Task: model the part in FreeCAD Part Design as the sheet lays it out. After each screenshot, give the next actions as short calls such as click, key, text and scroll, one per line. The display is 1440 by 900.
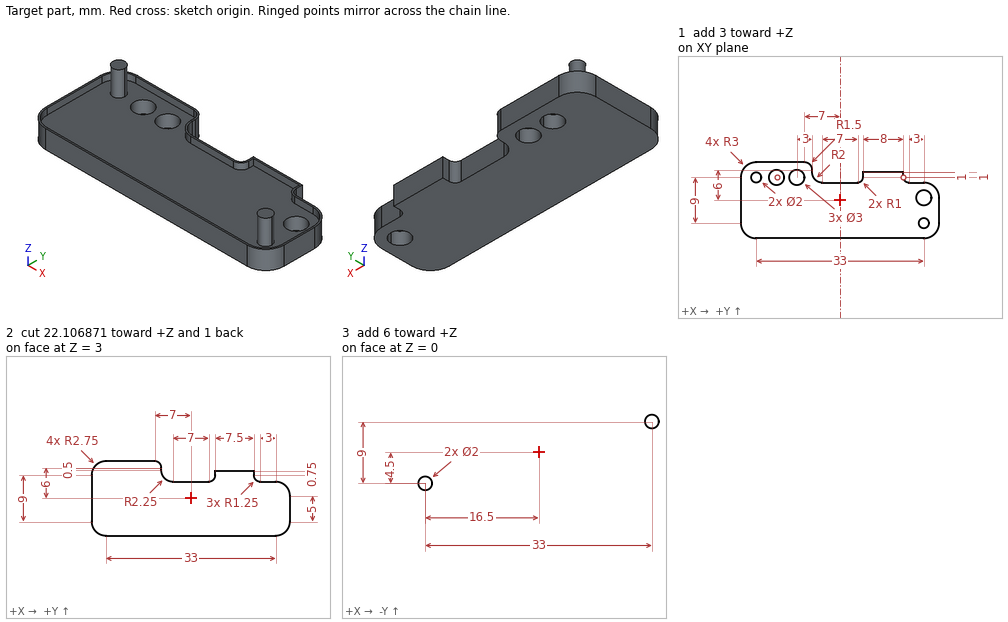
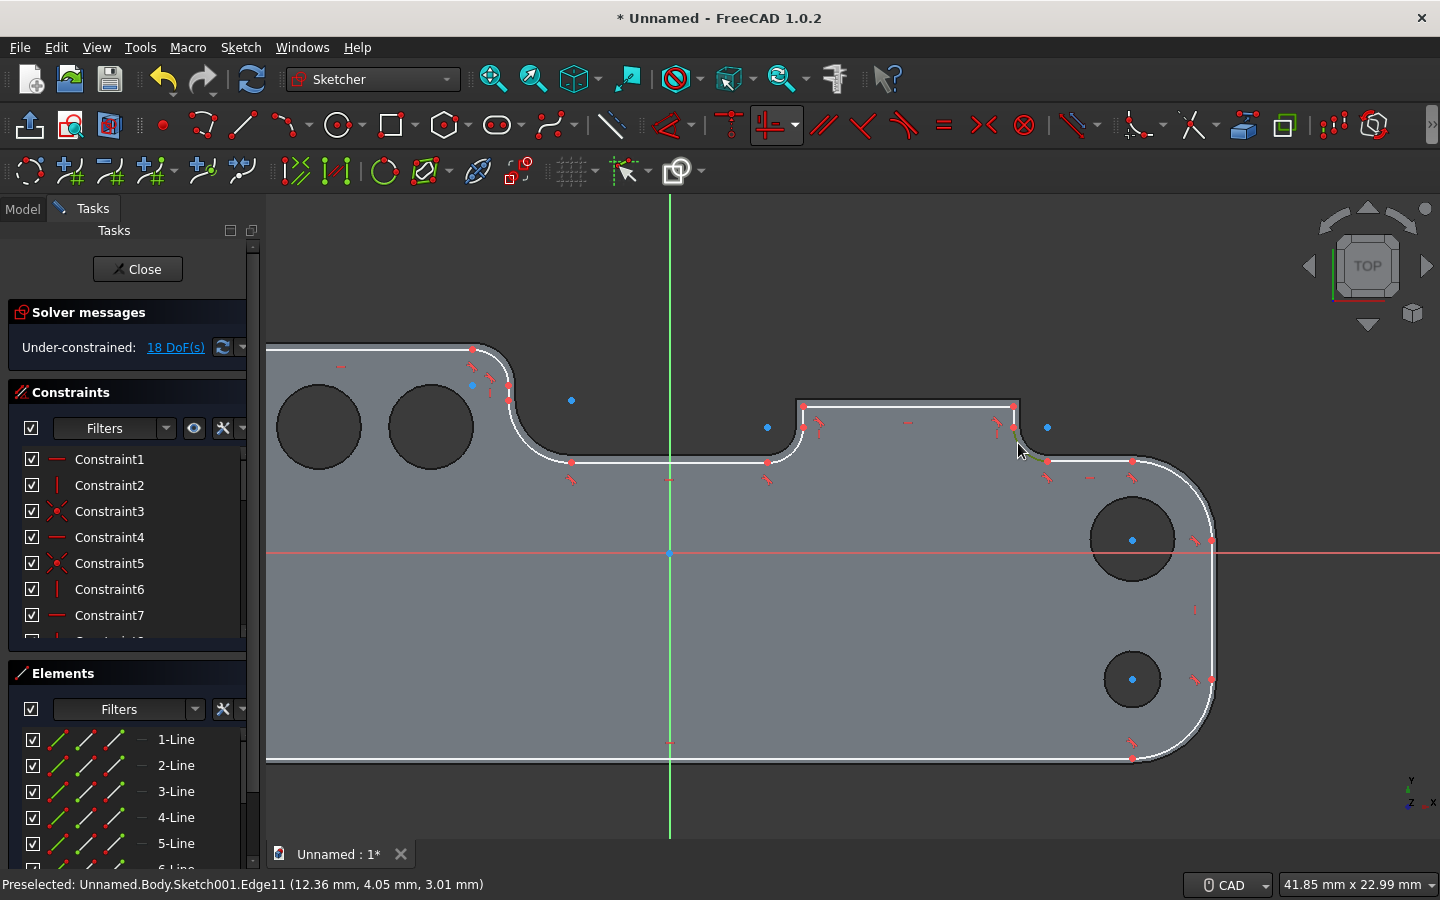
click(784, 459)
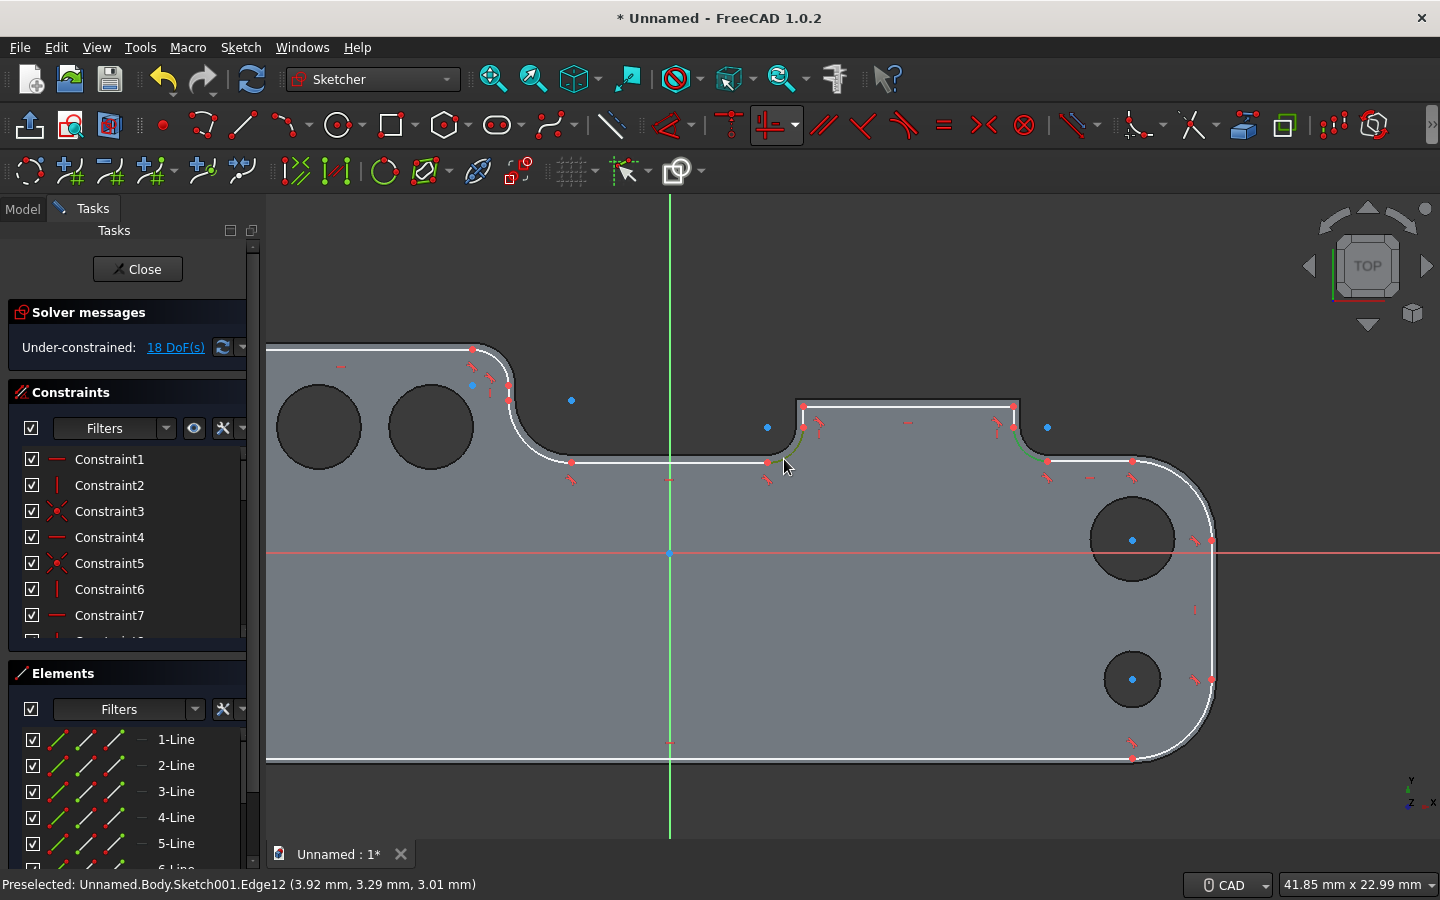
click(505, 370)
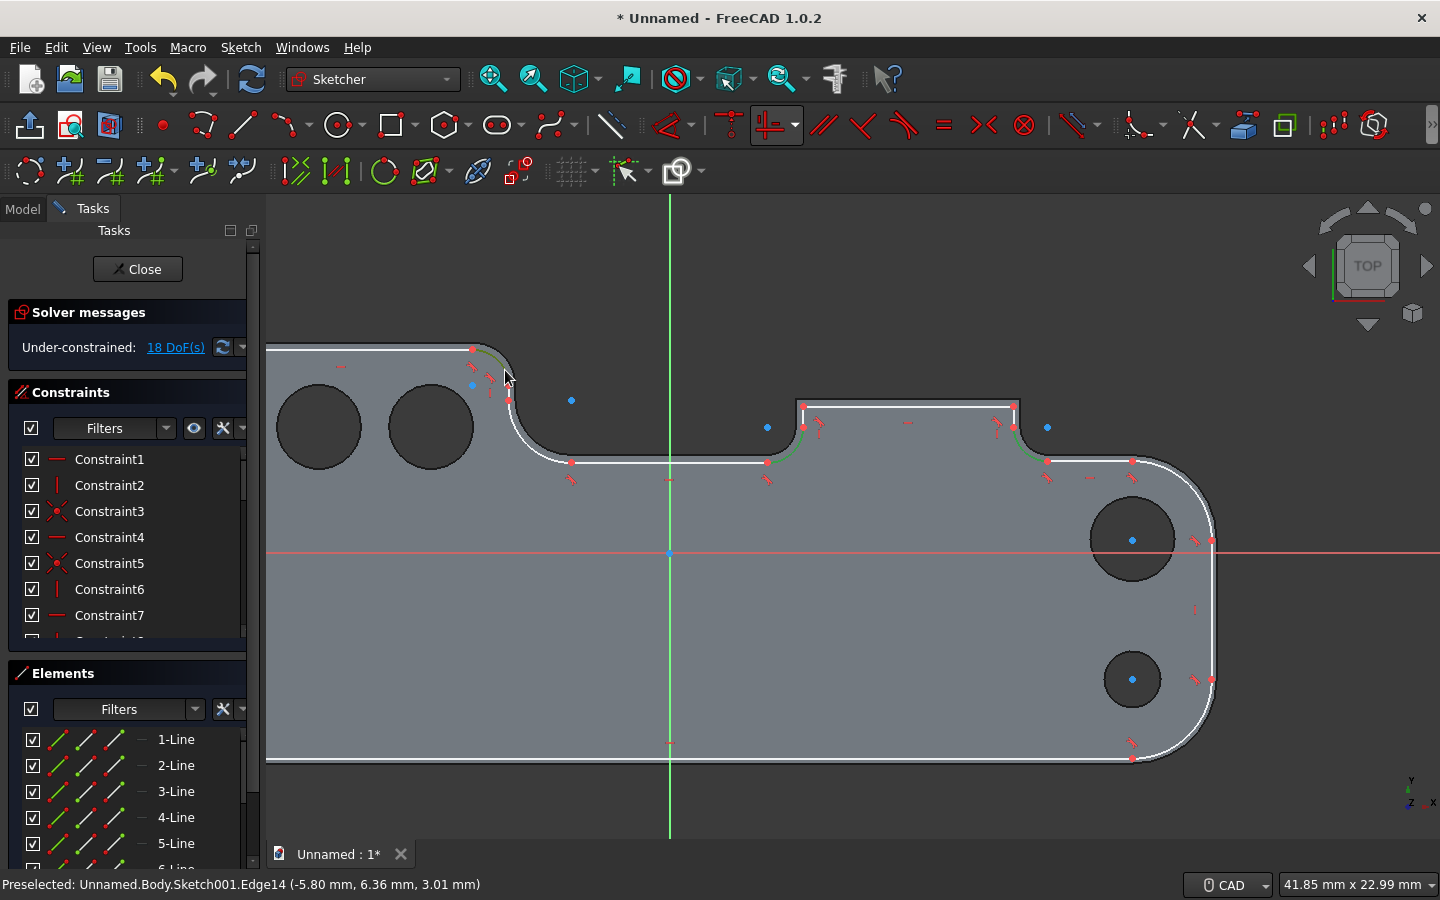
key(e)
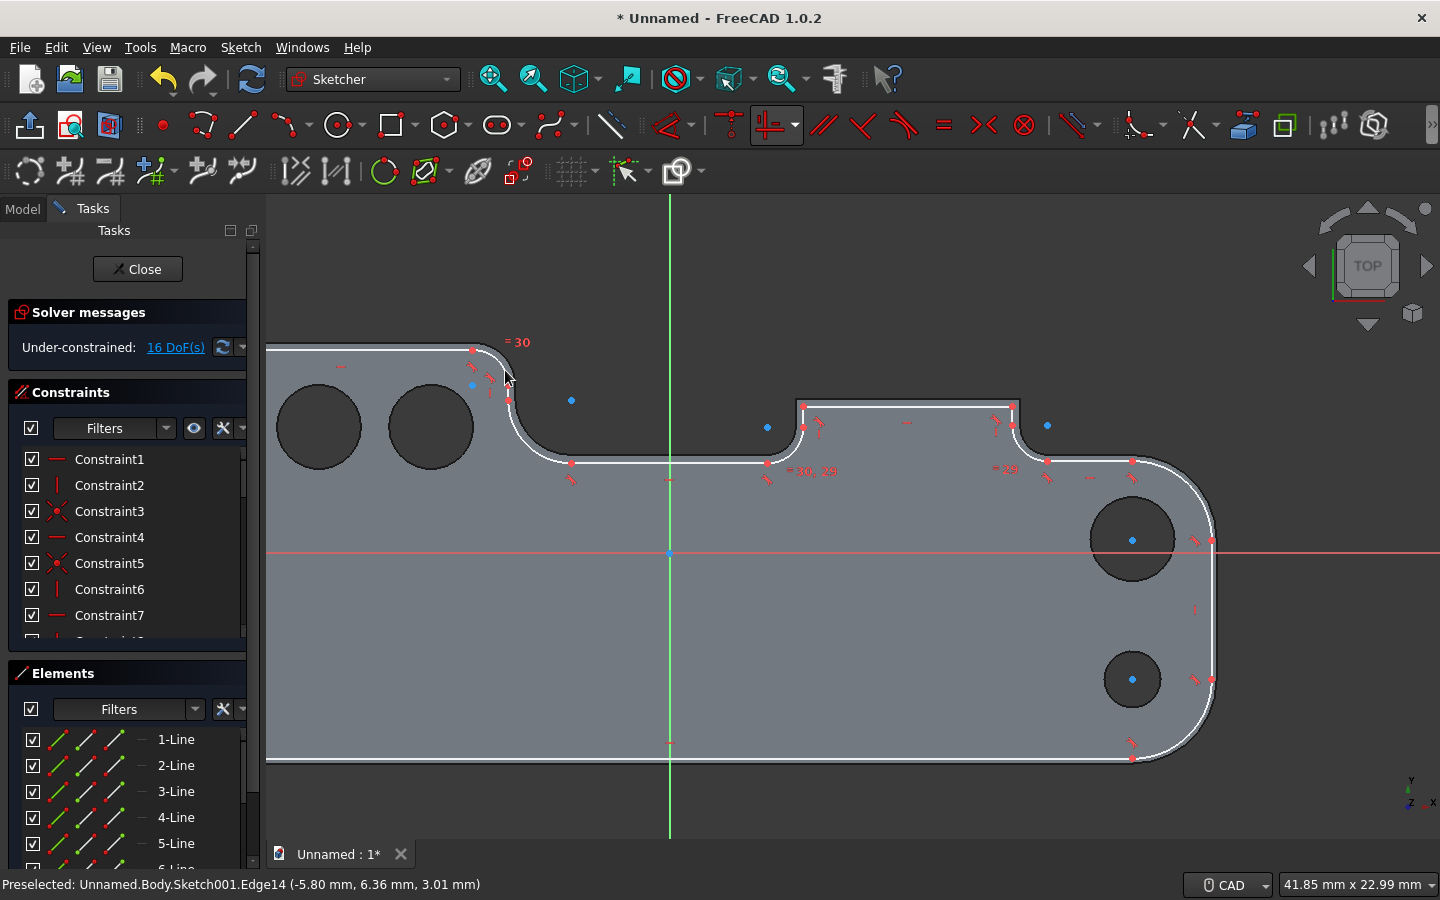
scroll(1018, 442, down, 2)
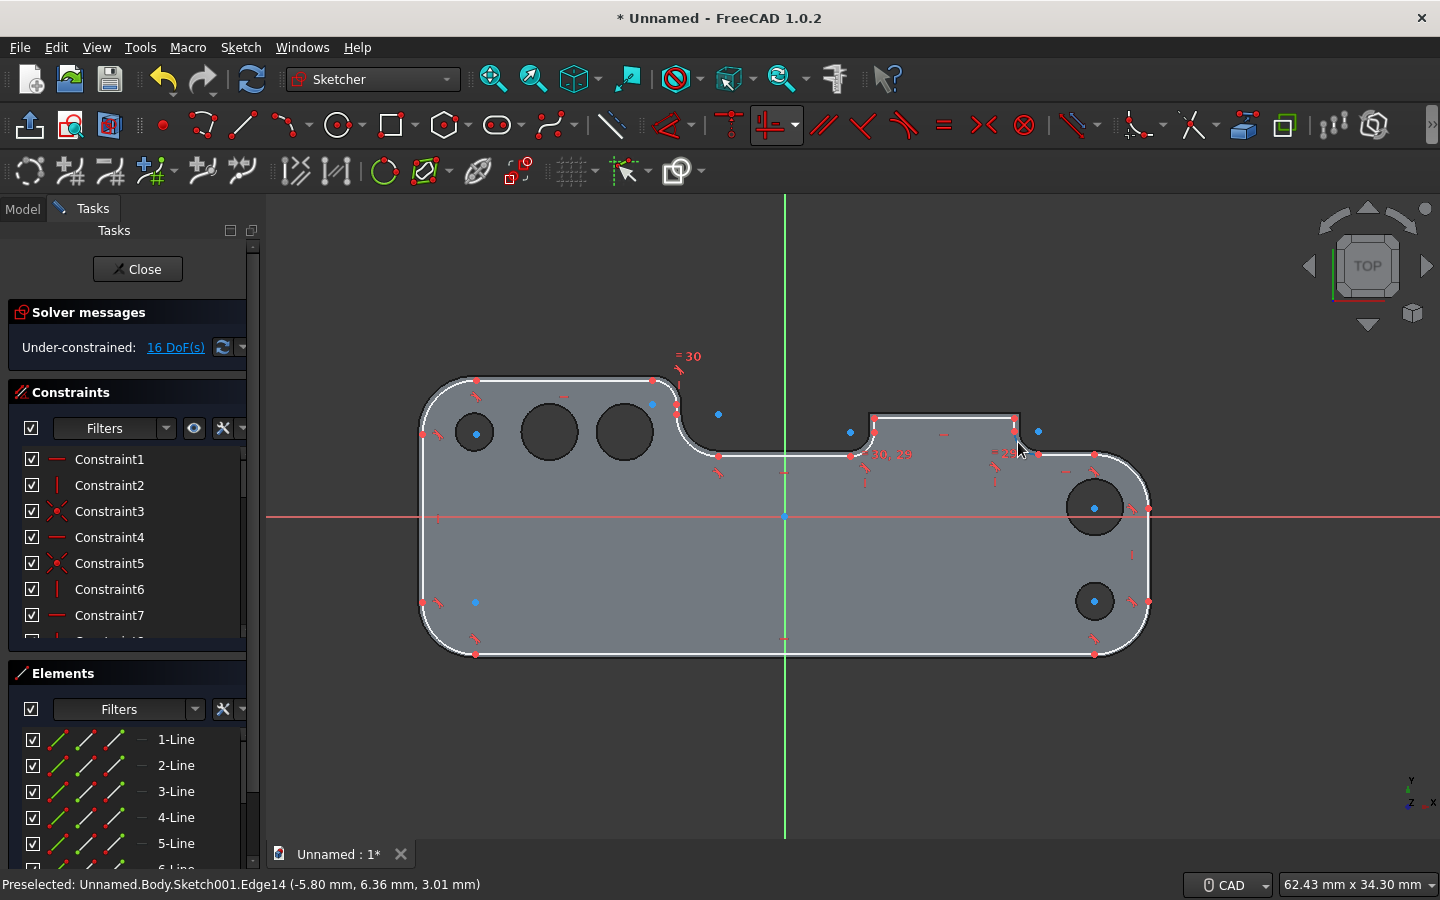
click(452, 386)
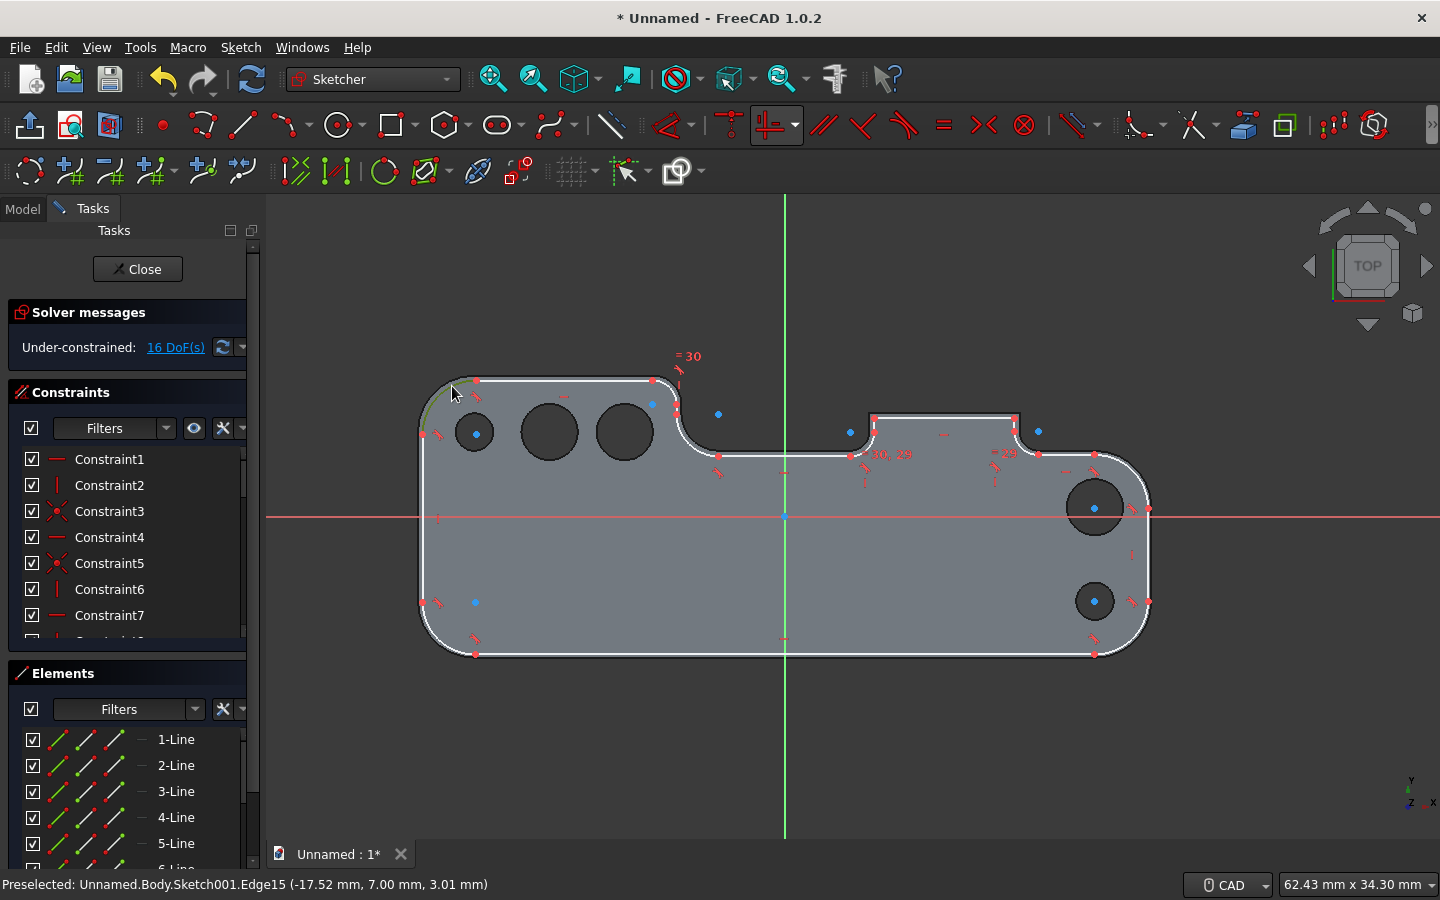
click(428, 626)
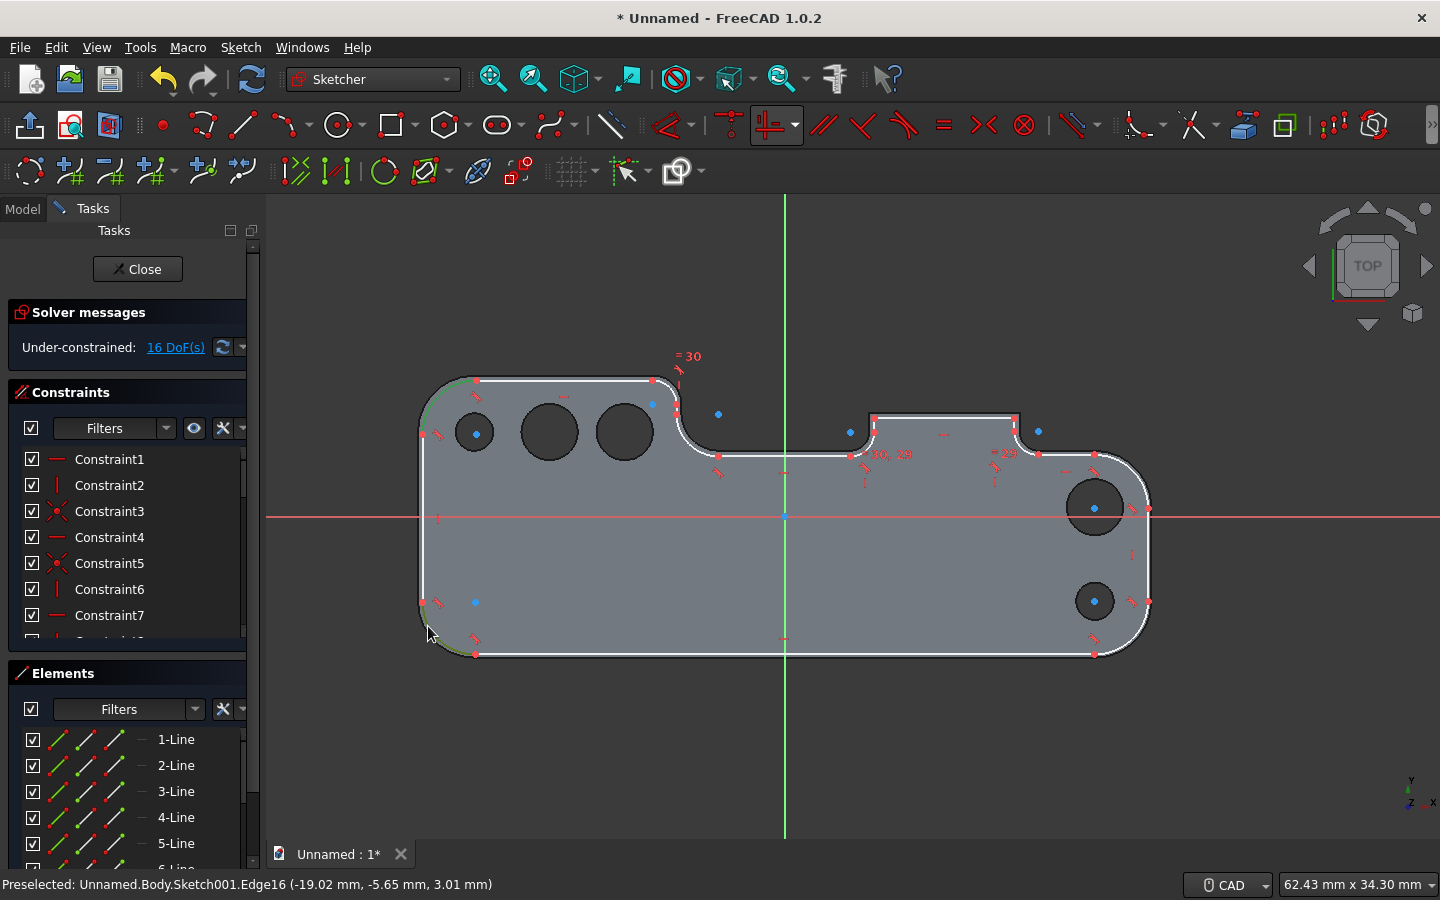
click(1119, 649)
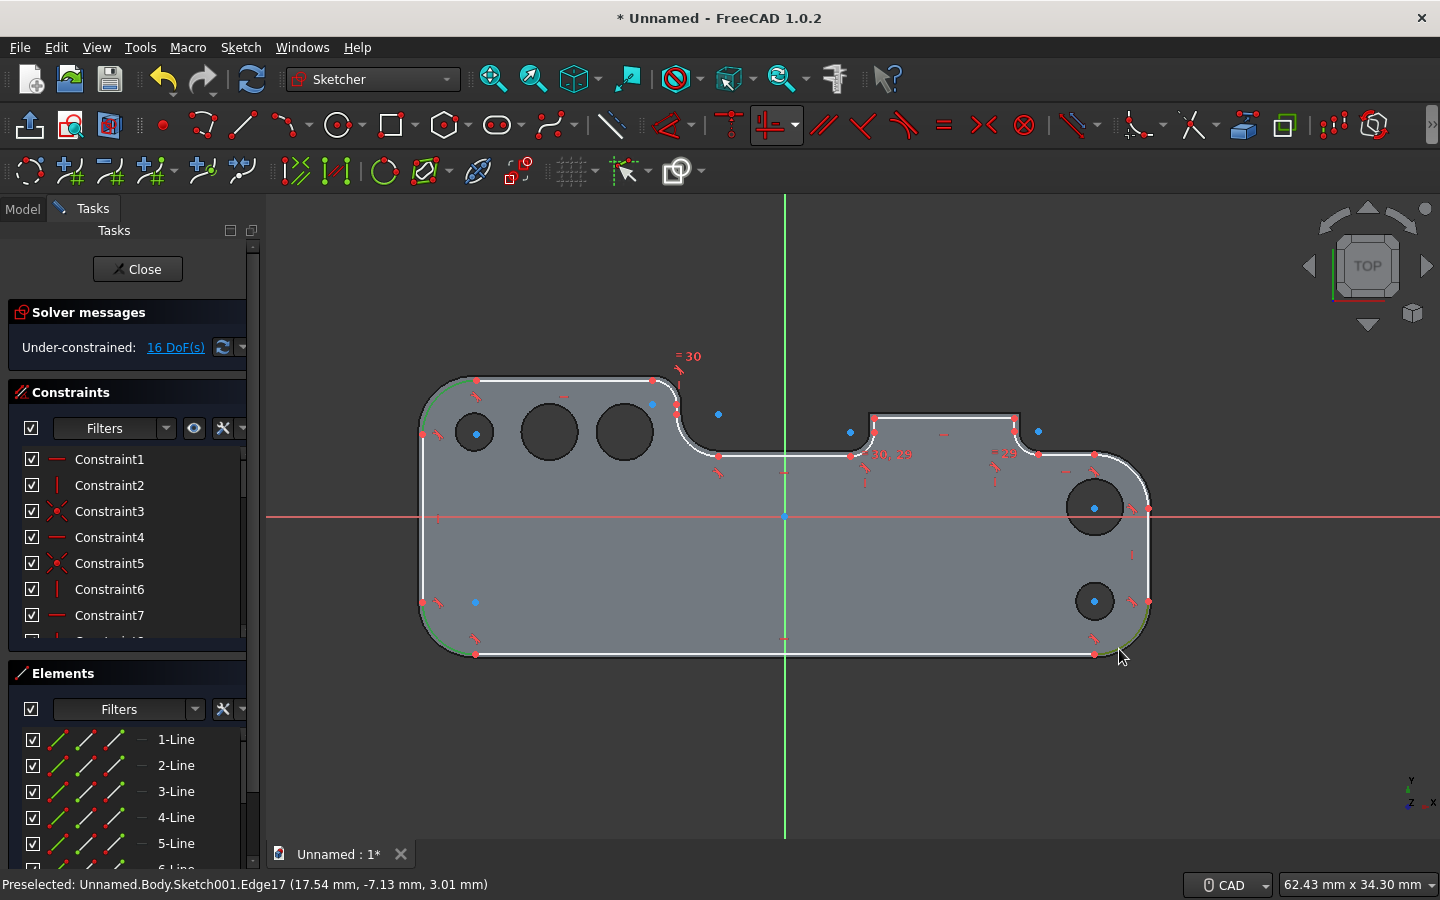
click(1142, 484)